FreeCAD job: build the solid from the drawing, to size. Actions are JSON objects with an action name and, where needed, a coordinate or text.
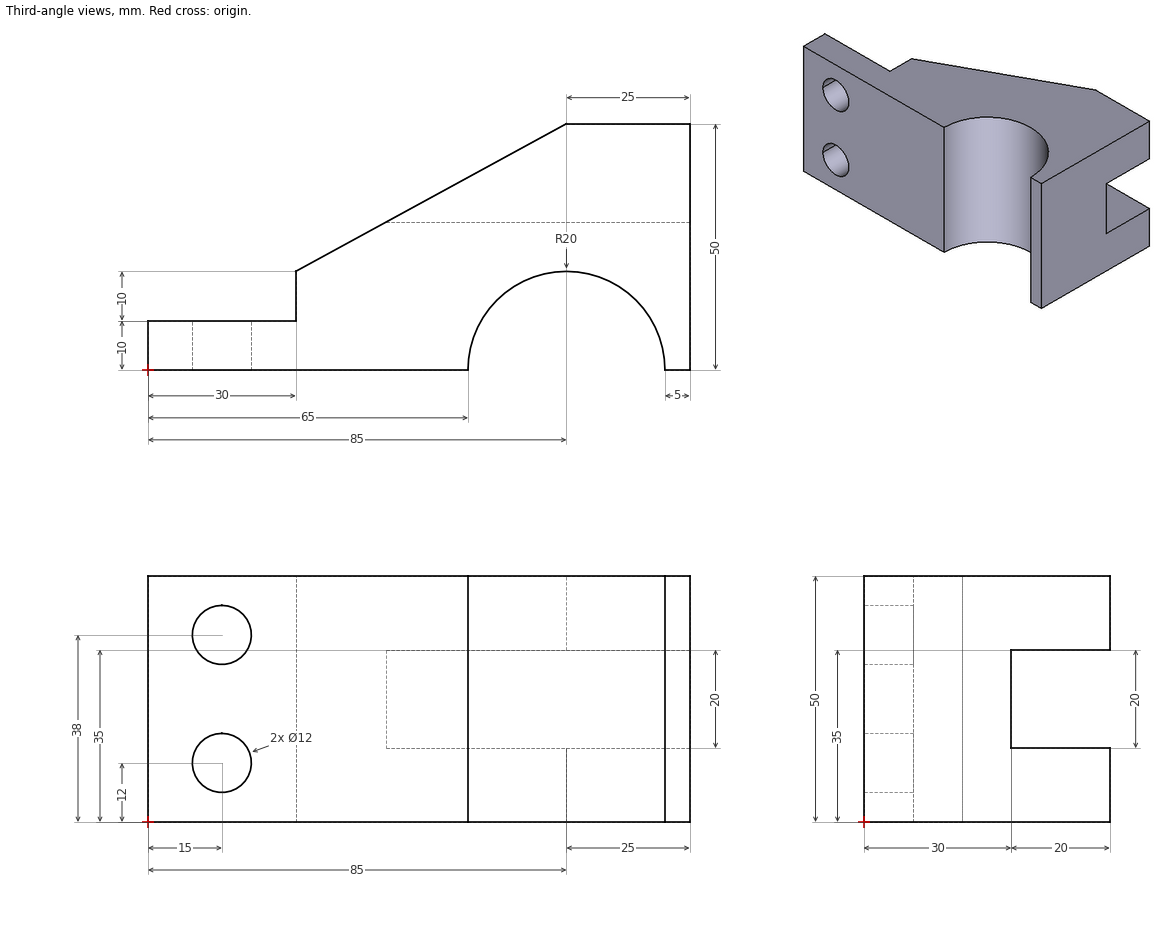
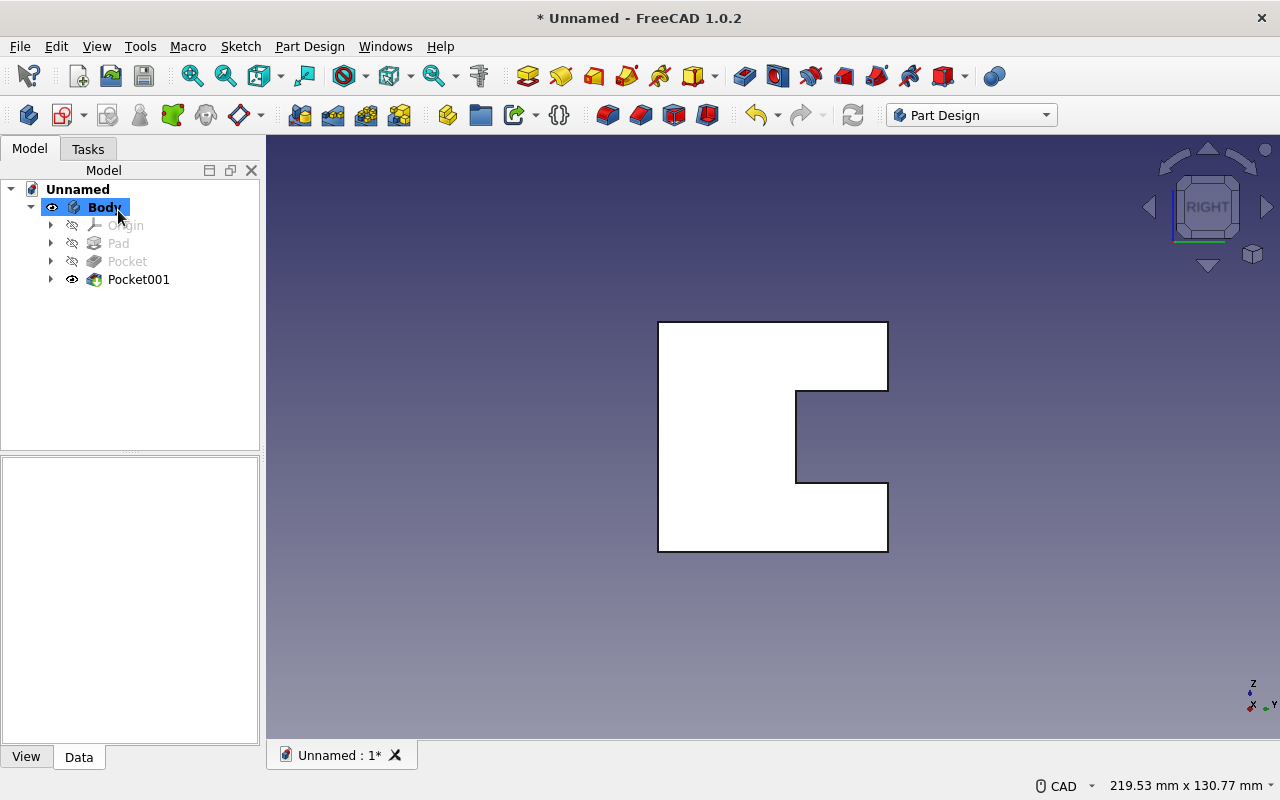
{"action": "left_click", "coordinate": [193, 76]}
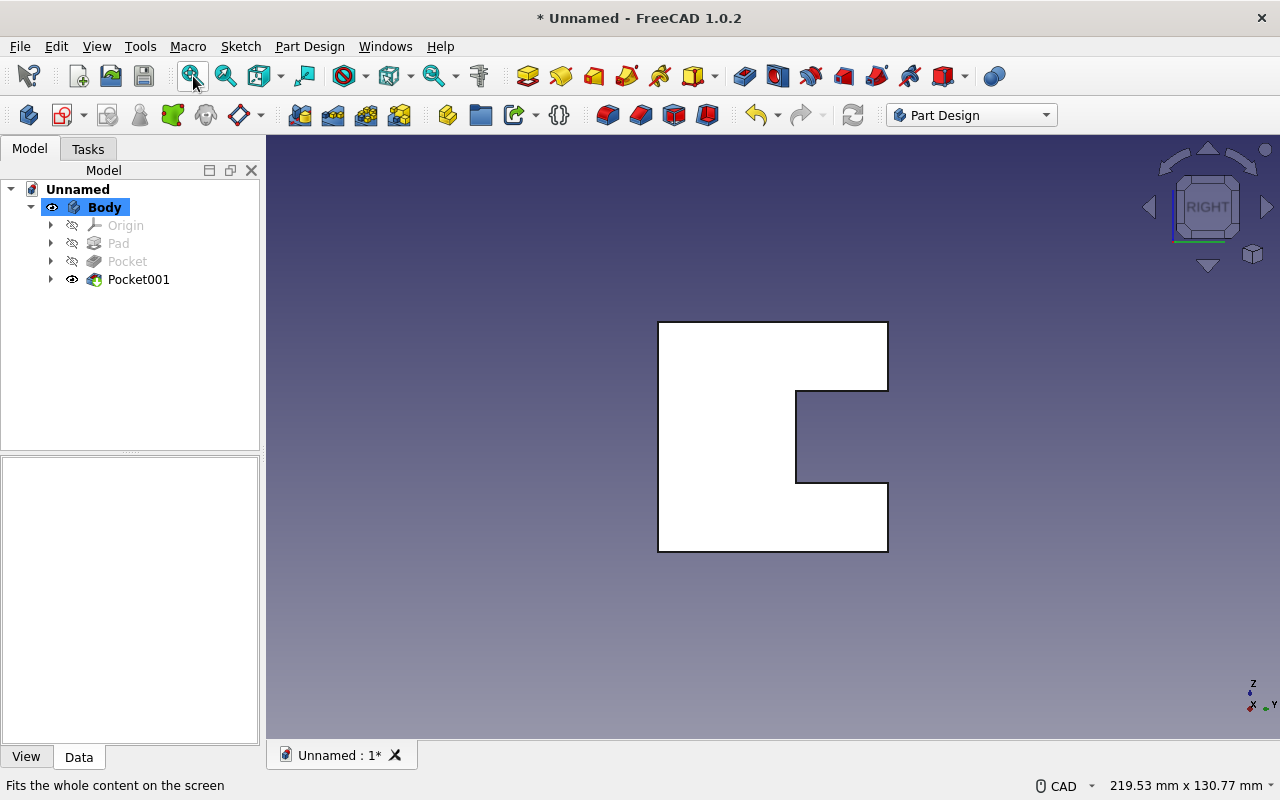
{"action": "key", "text": "4"}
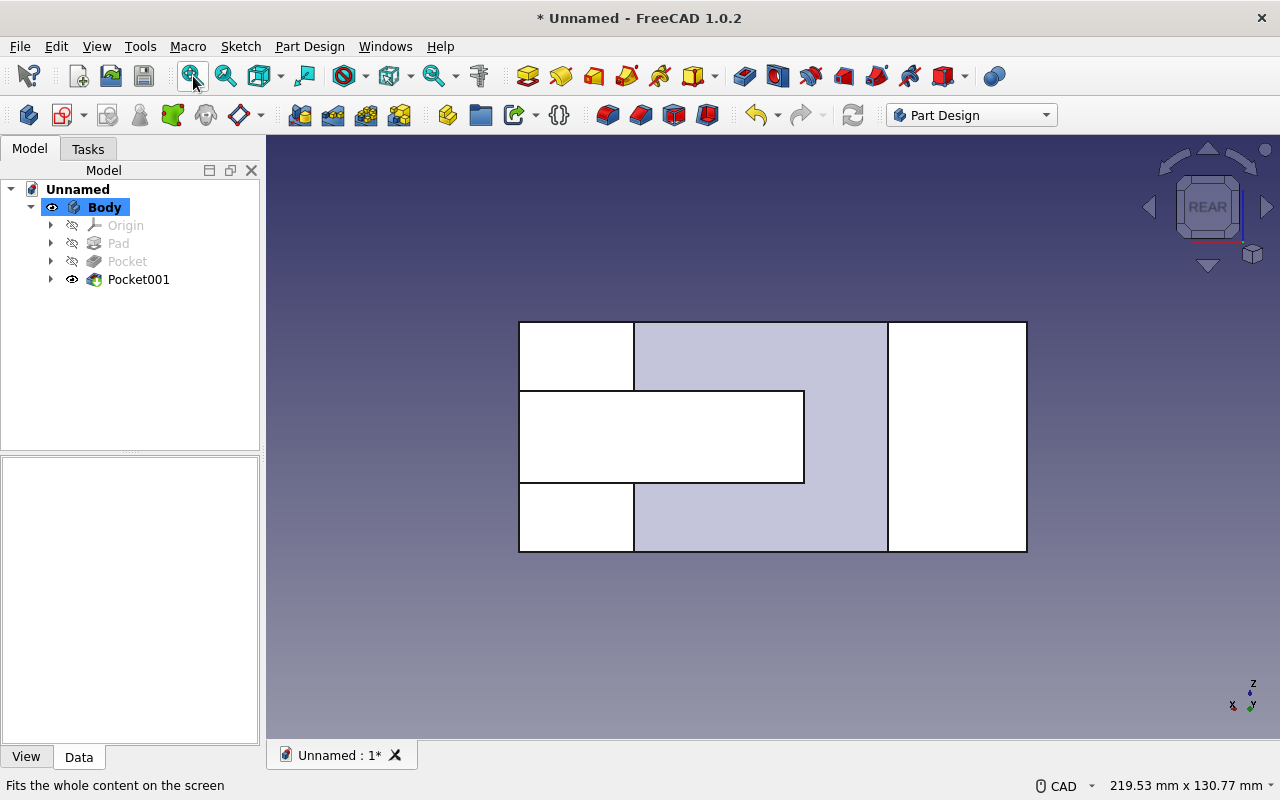
{"action": "left_click", "coordinate": [958, 403]}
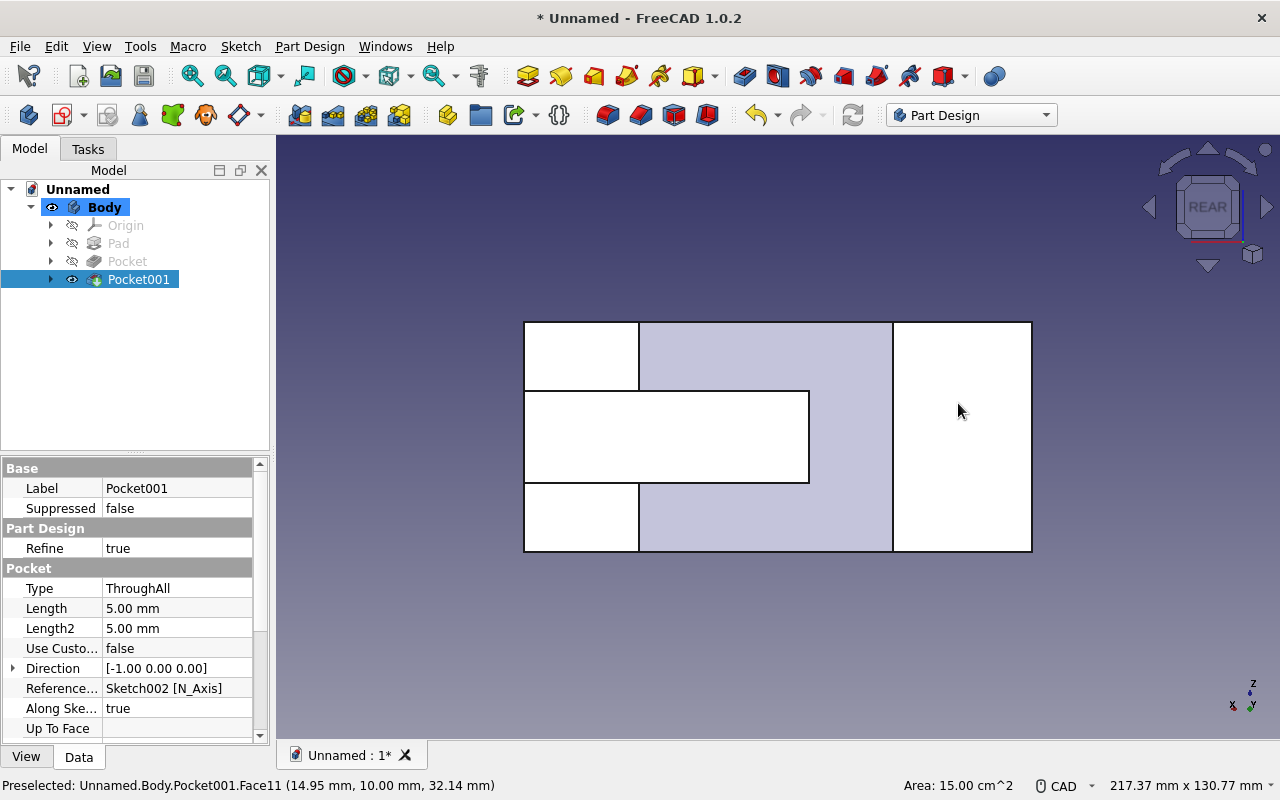
{"action": "left_click", "coordinate": [62, 116]}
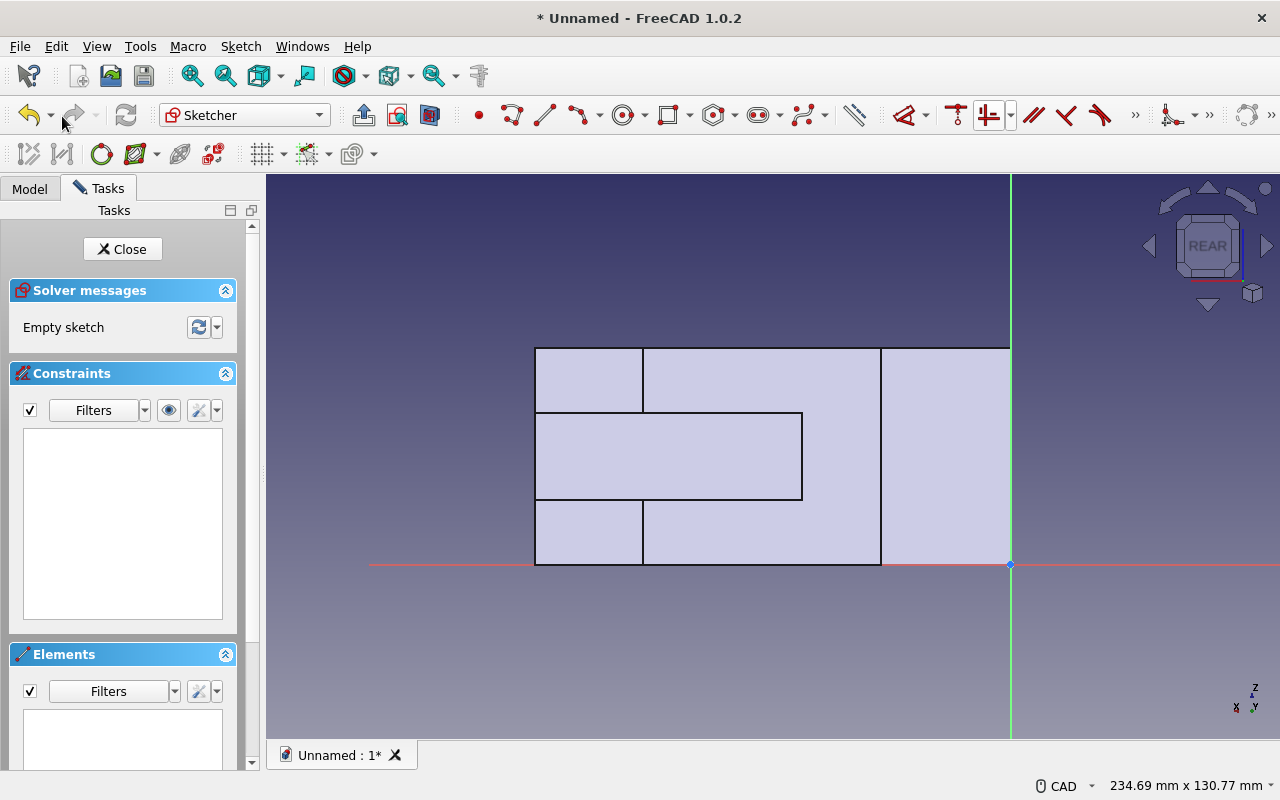
{"action": "scroll", "coordinate": [1115, 485], "scroll_direction": "up", "scroll_amount": 3}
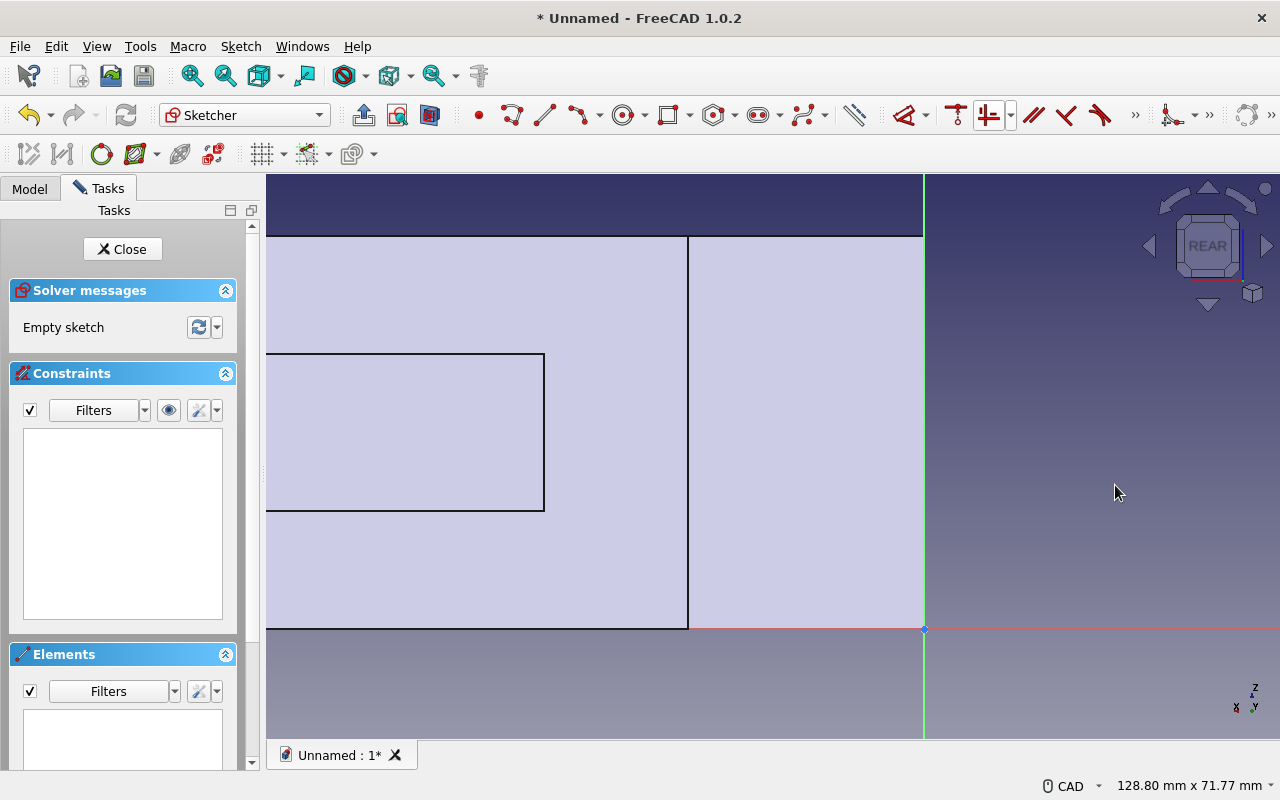
{"action": "left_click", "coordinate": [622, 116]}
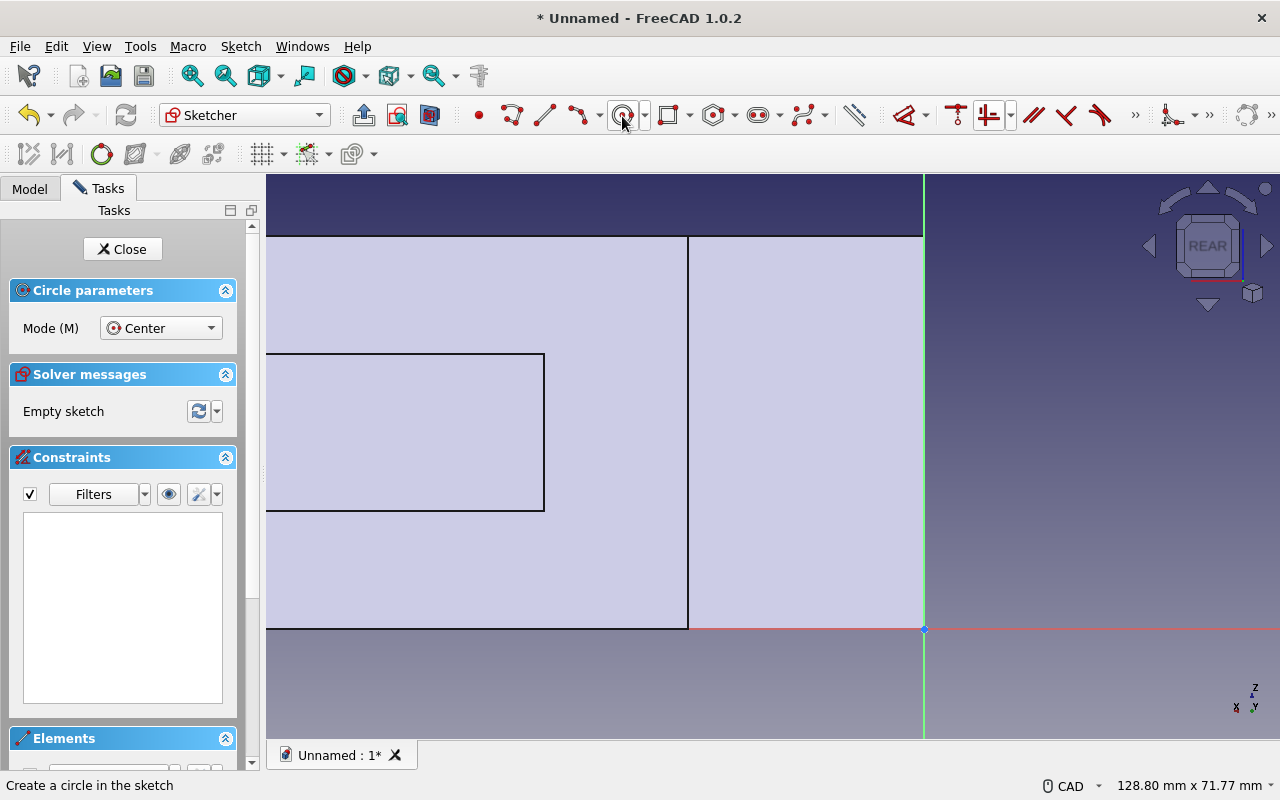
{"action": "left_click", "coordinate": [806, 535]}
{"action": "left_click", "coordinate": [839, 502]}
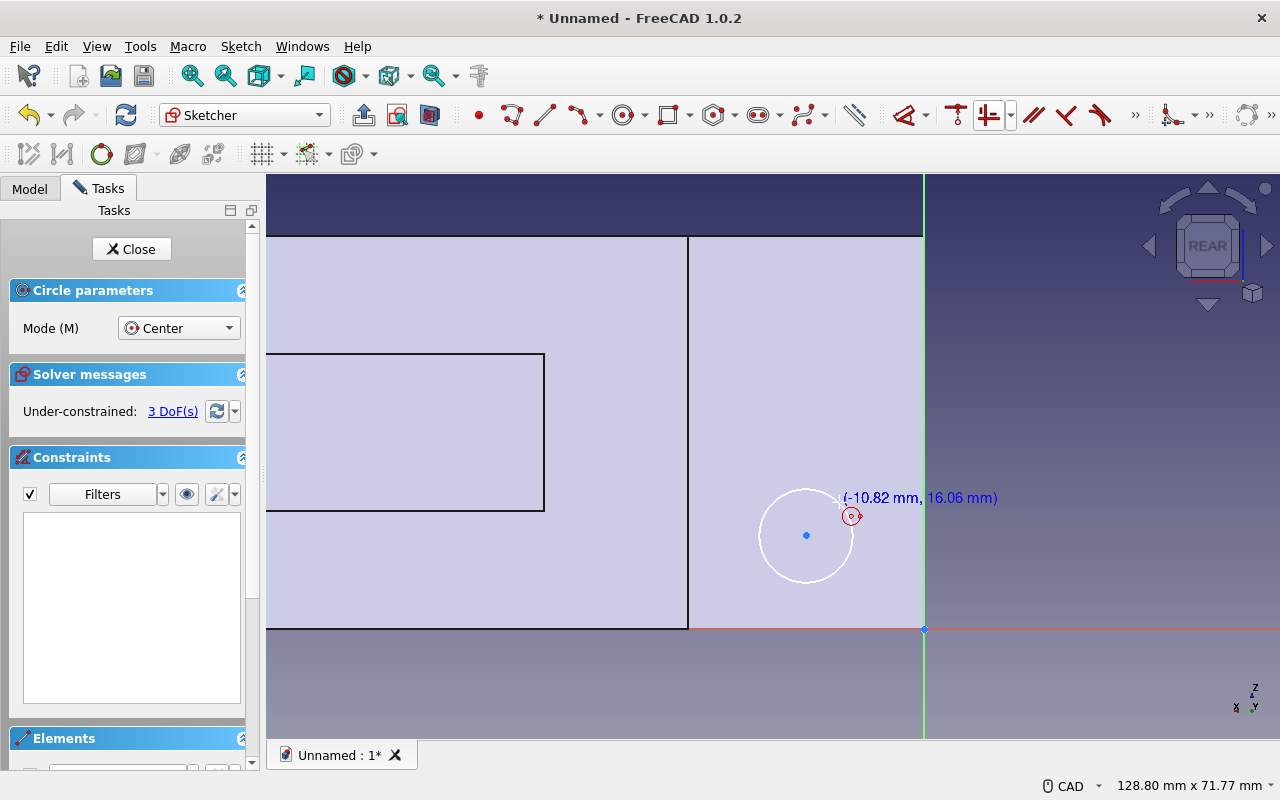
{"action": "left_click", "coordinate": [806, 330]}
{"action": "left_click", "coordinate": [839, 297]}
{"action": "key", "text": "Escape"}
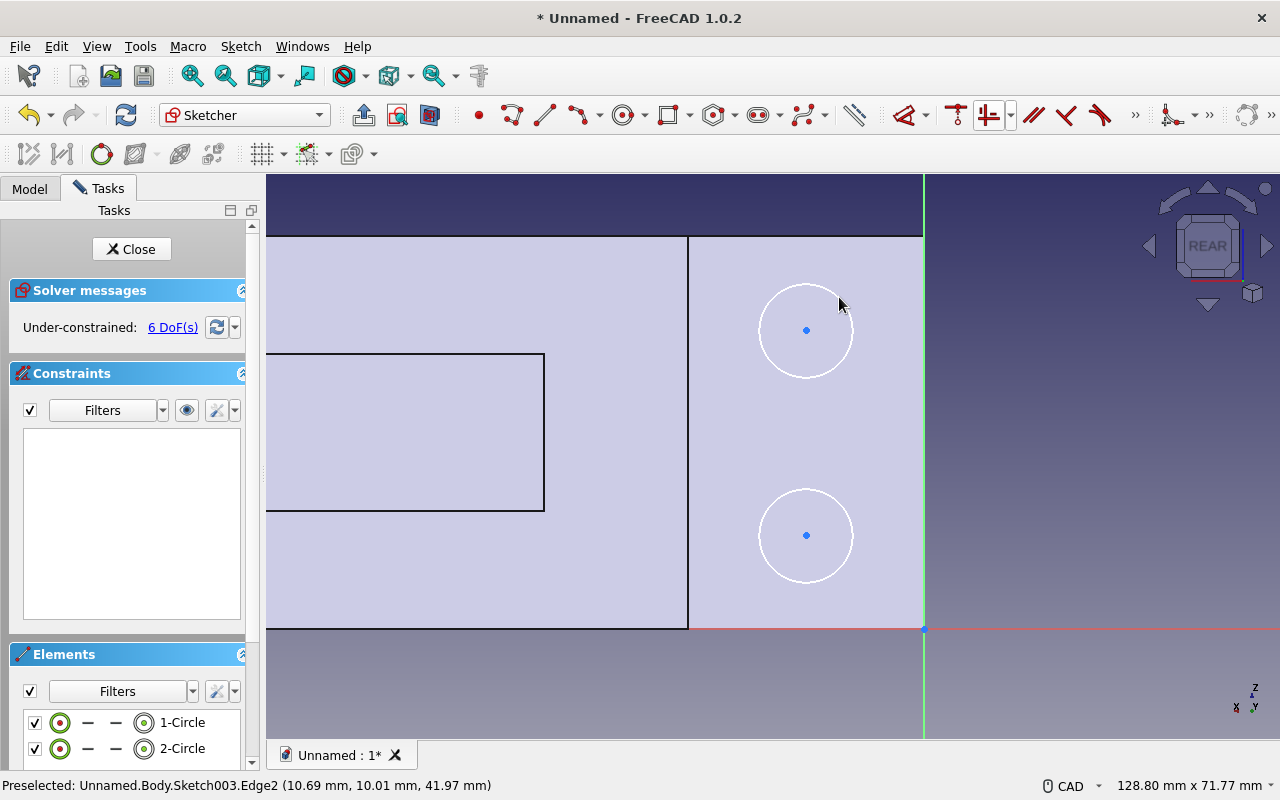
{"action": "left_click", "coordinate": [839, 503]}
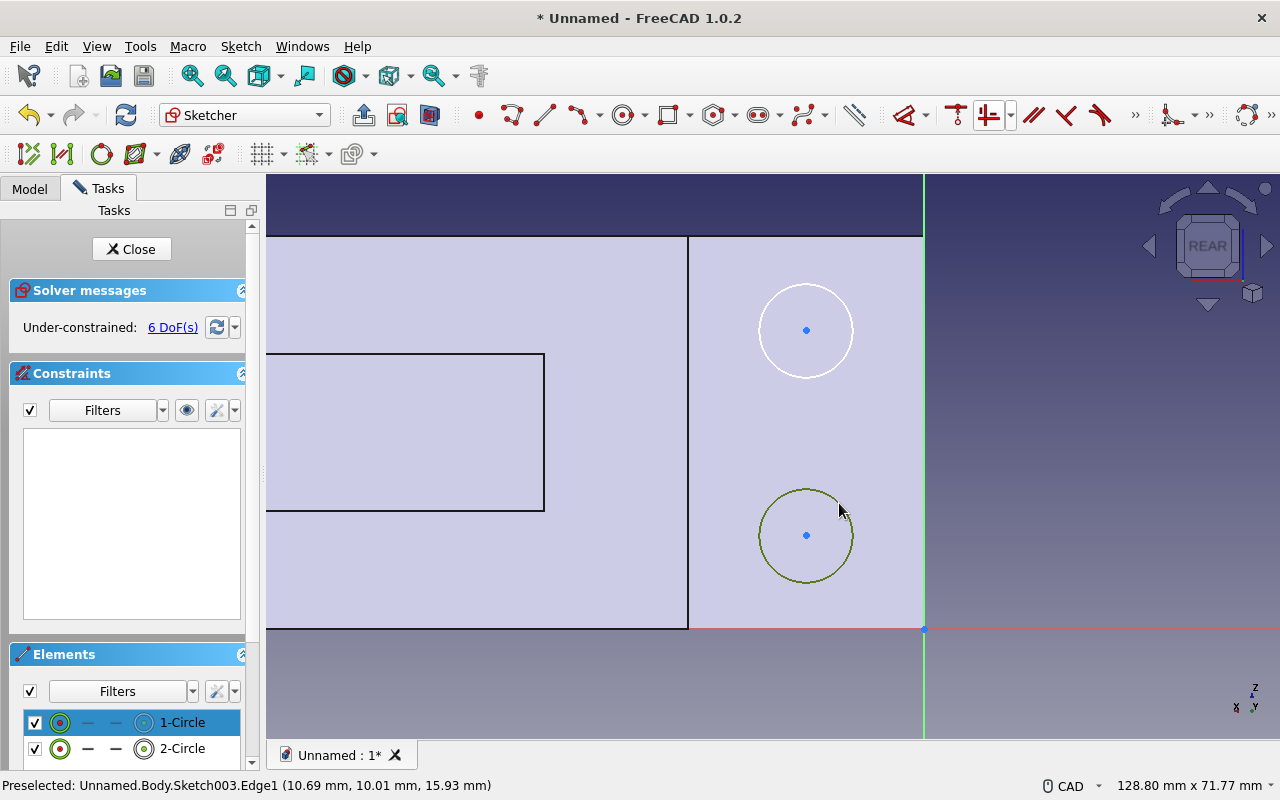
{"action": "left_click", "coordinate": [839, 298]}